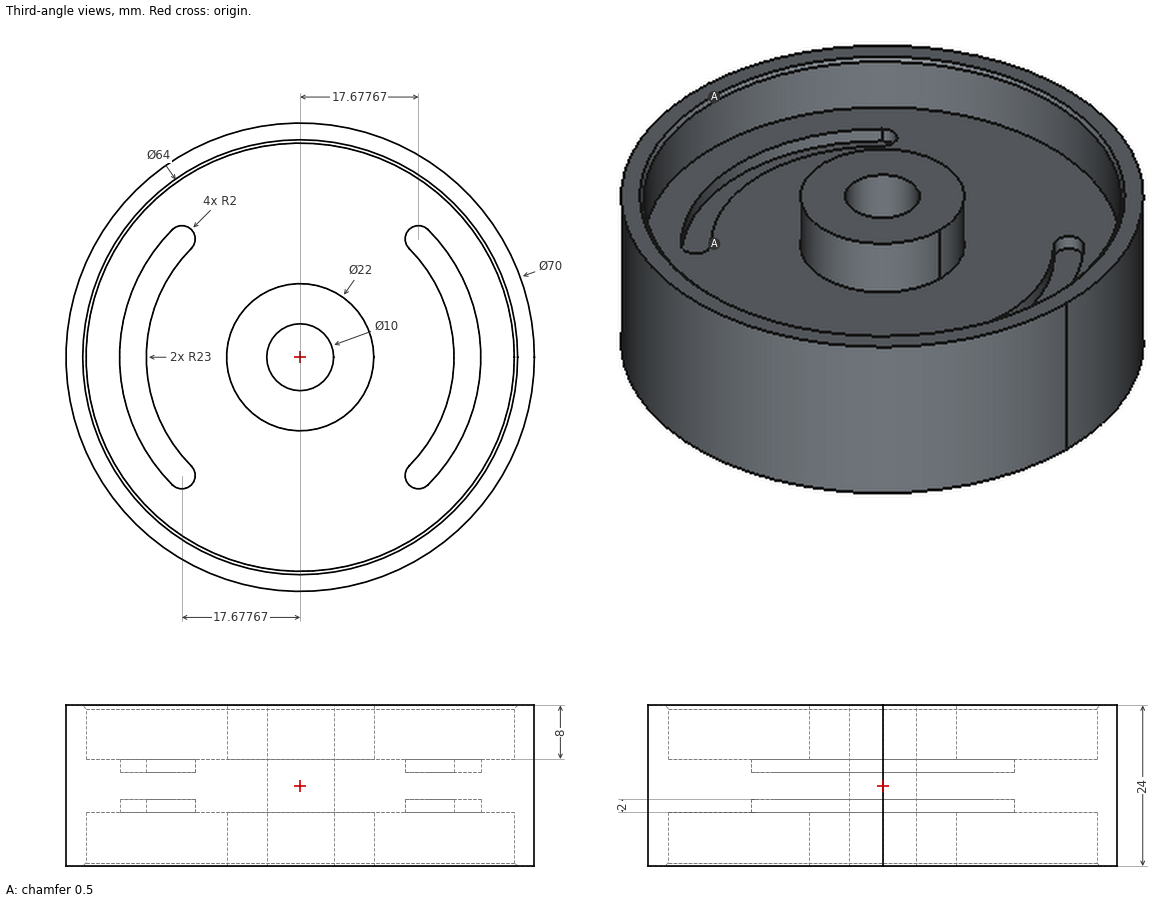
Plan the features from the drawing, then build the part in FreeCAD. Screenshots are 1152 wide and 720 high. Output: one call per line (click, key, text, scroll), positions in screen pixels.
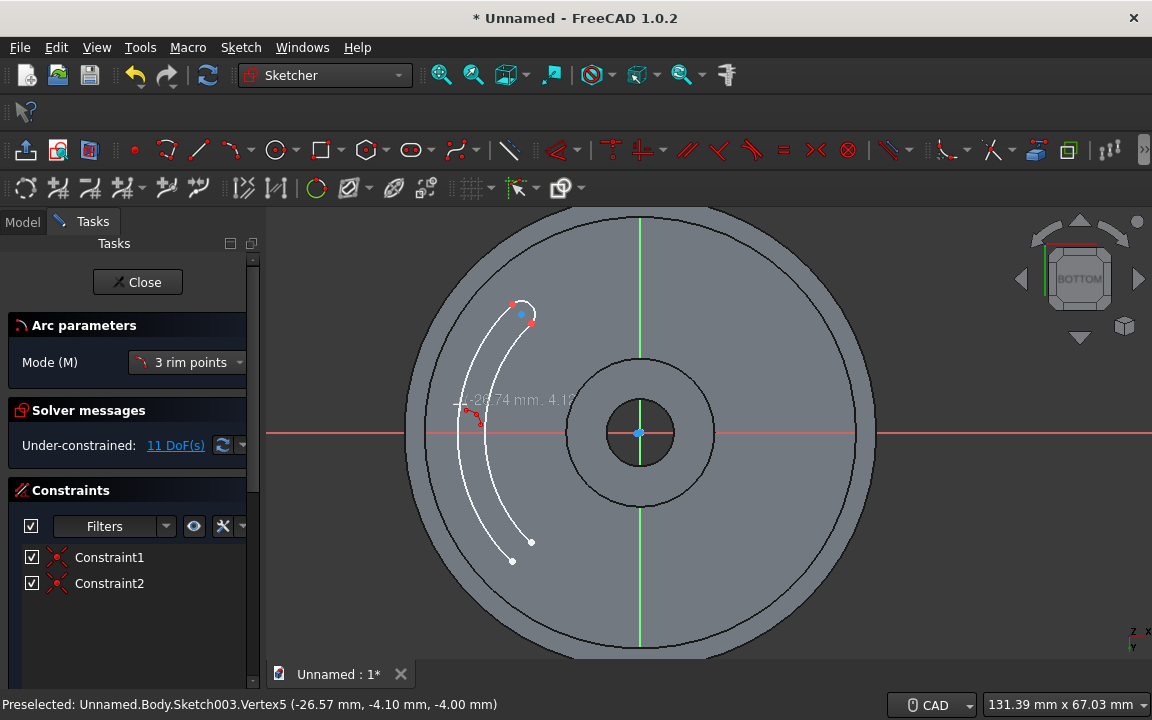
click(512, 562)
click(531, 543)
click(531, 561)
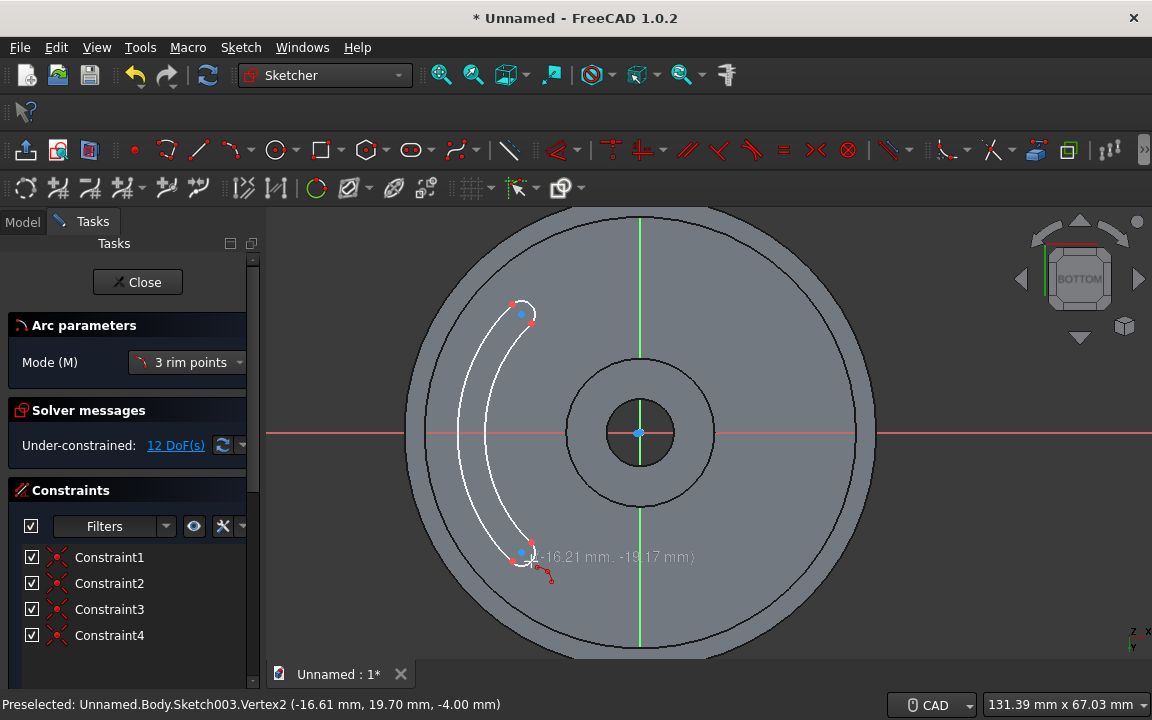
click(750, 323)
click(750, 542)
click(793, 457)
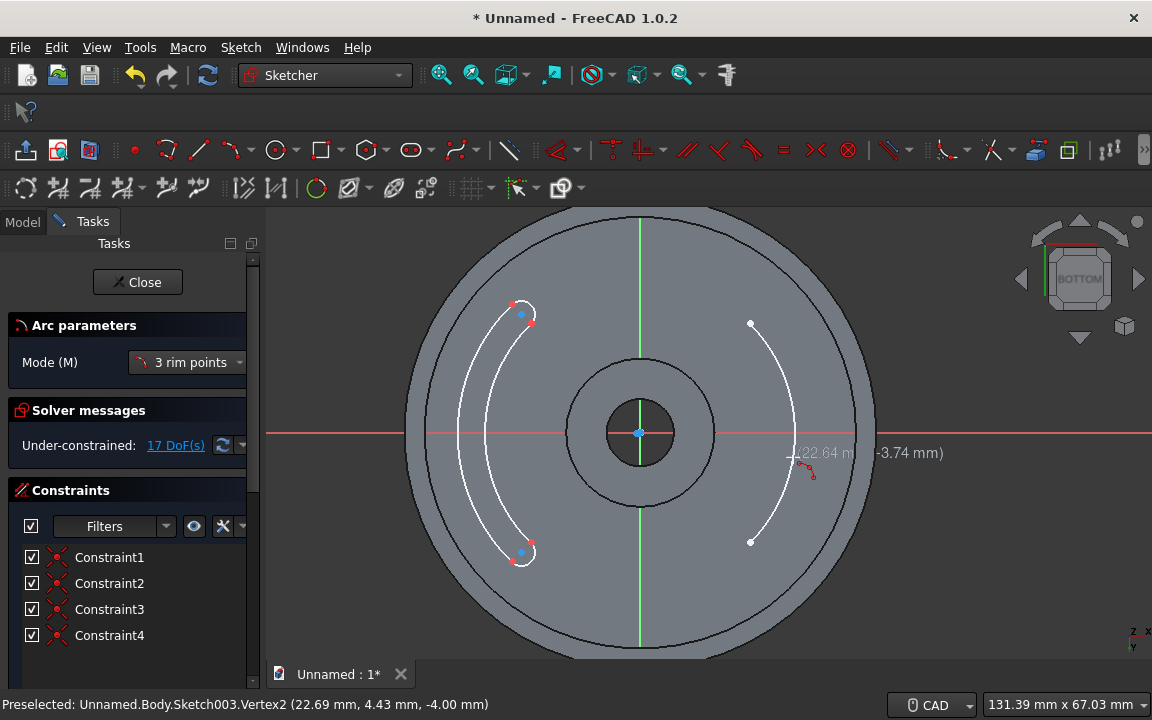
click(750, 543)
click(769, 561)
click(750, 561)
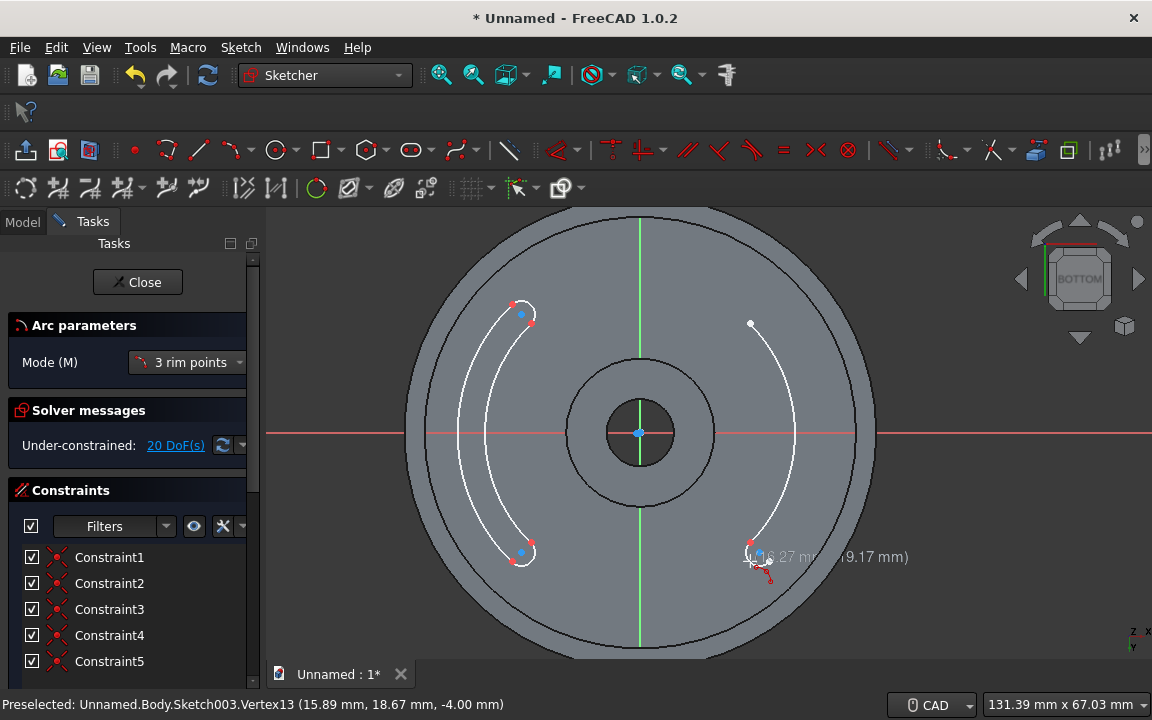
click(769, 562)
click(769, 304)
click(820, 461)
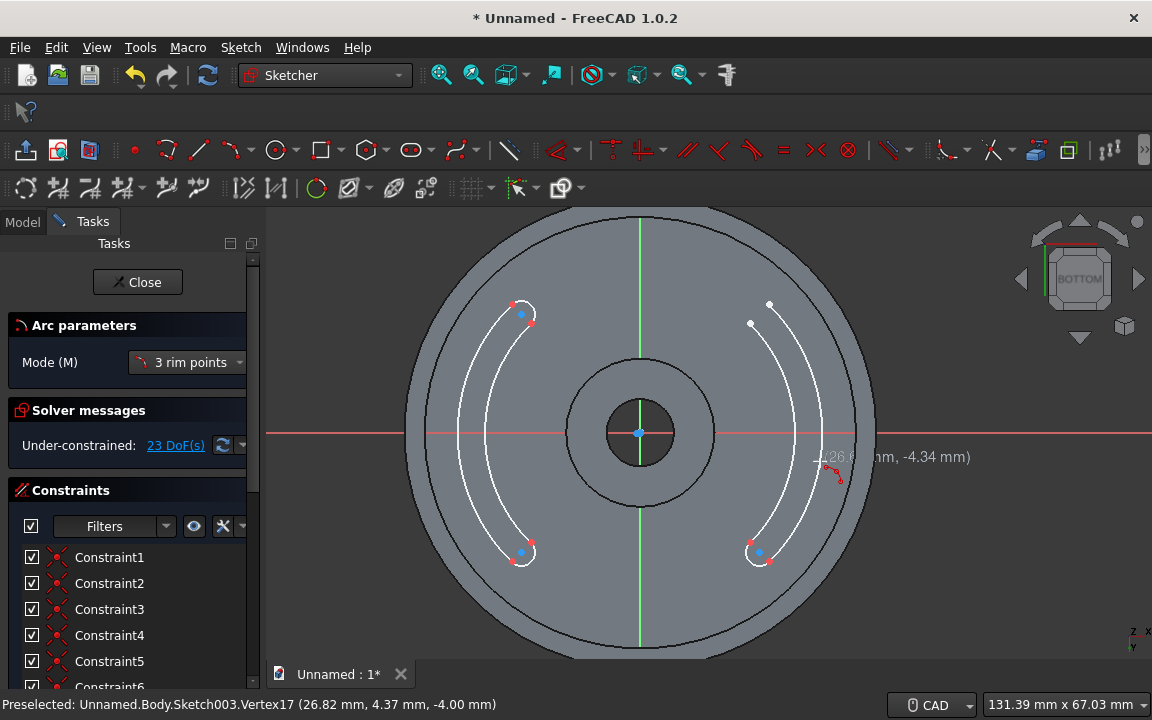
click(769, 305)
click(750, 324)
click(750, 304)
key(Escape)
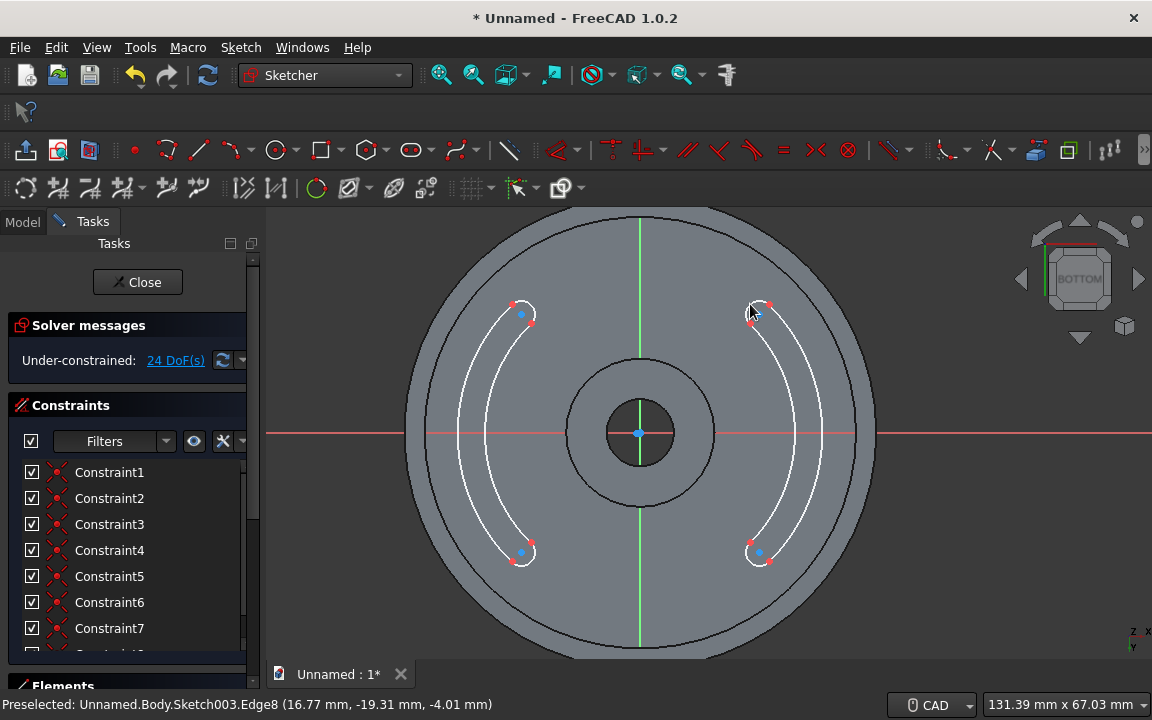
click(493, 386)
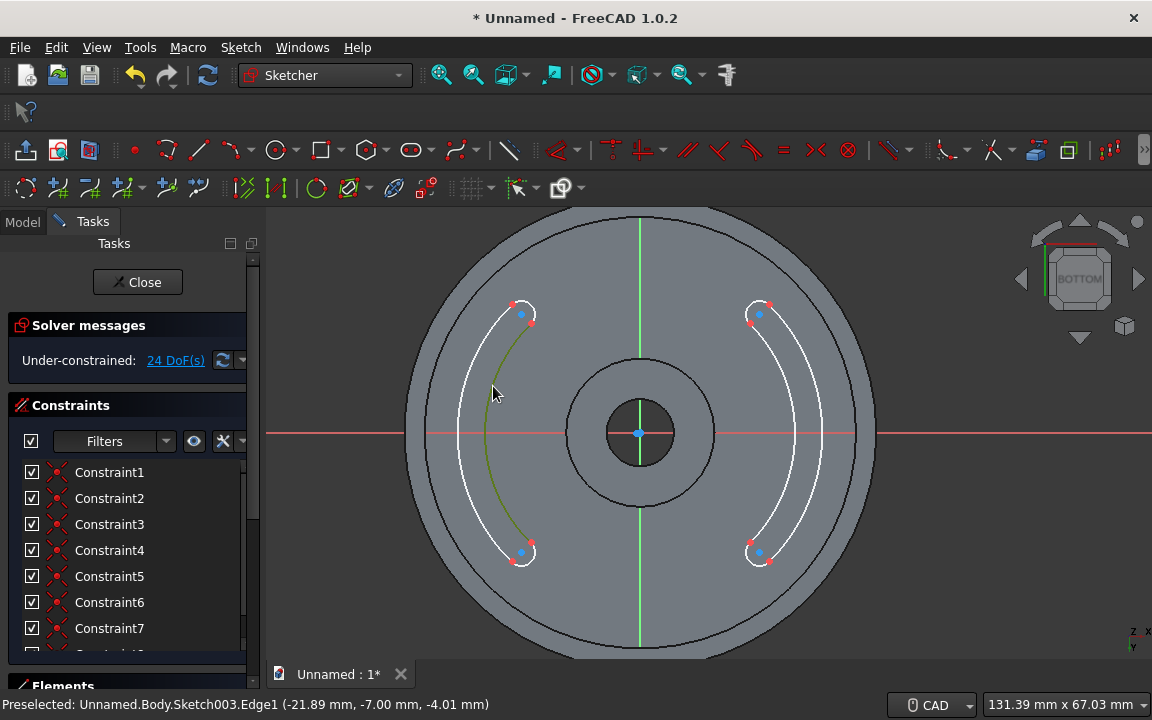
click(535, 312)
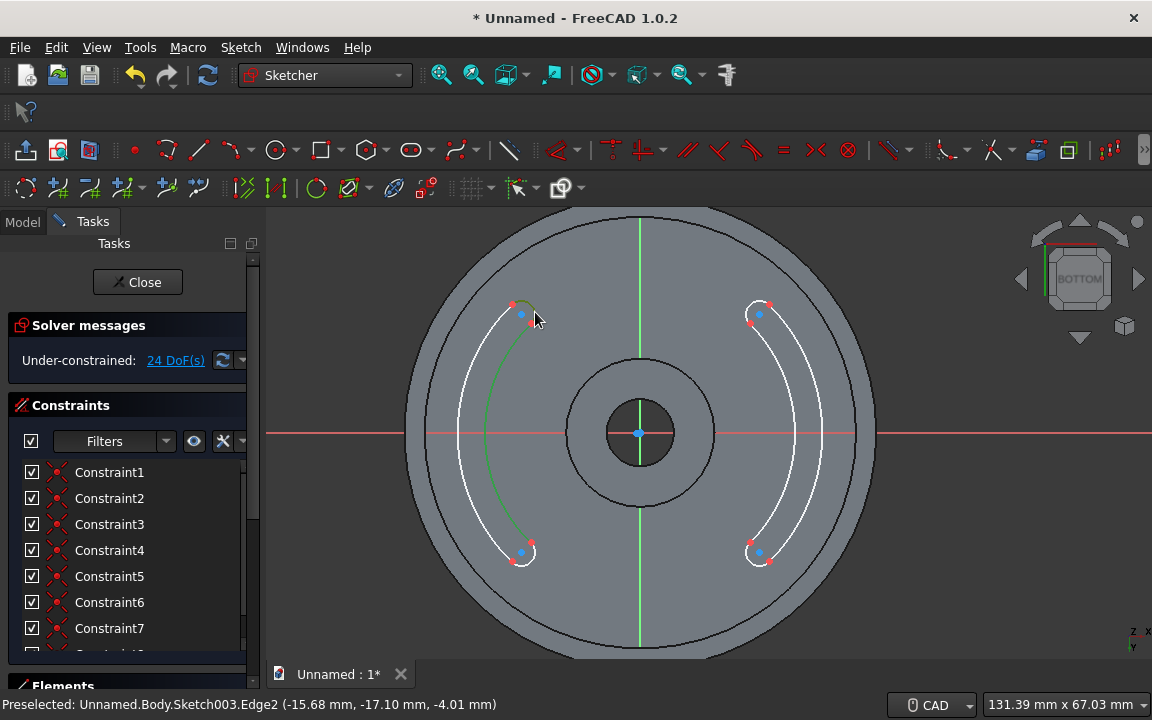
key(t)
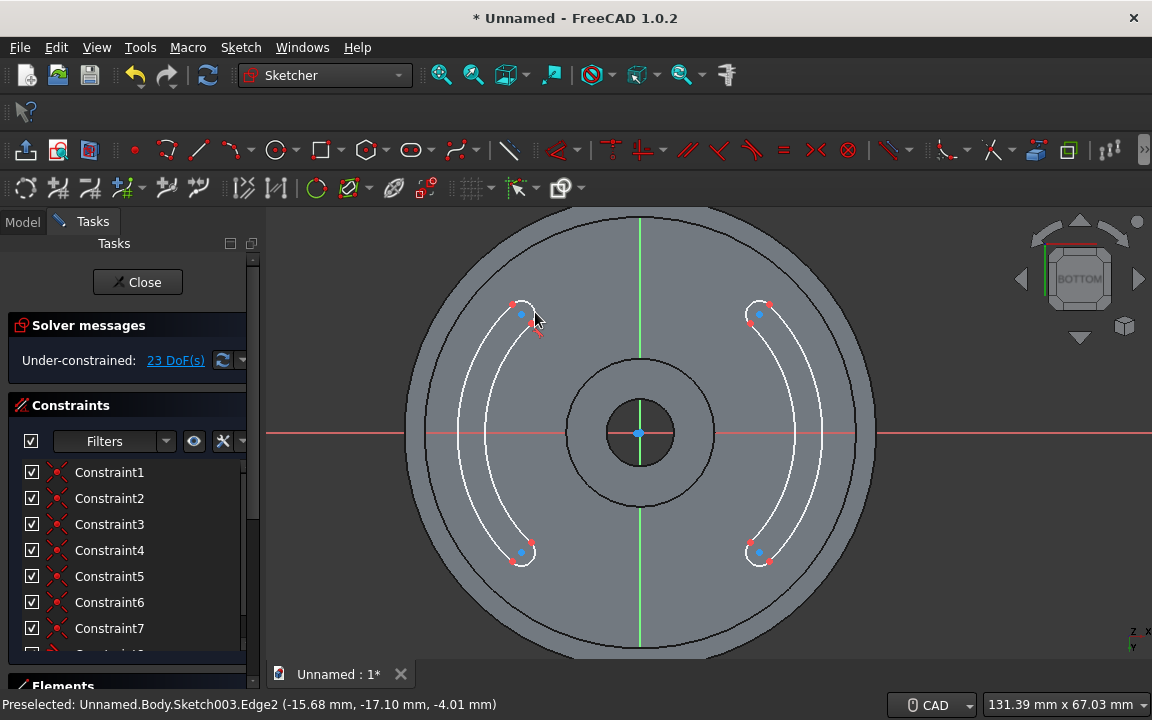
click(493, 386)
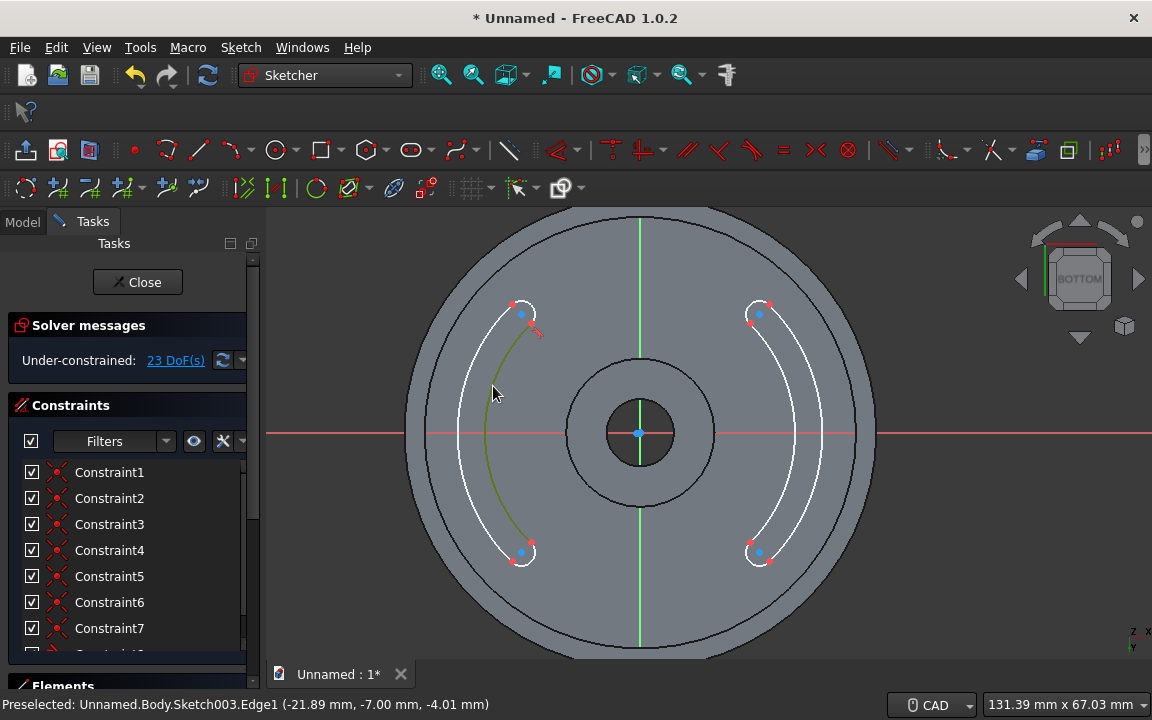
click(524, 566)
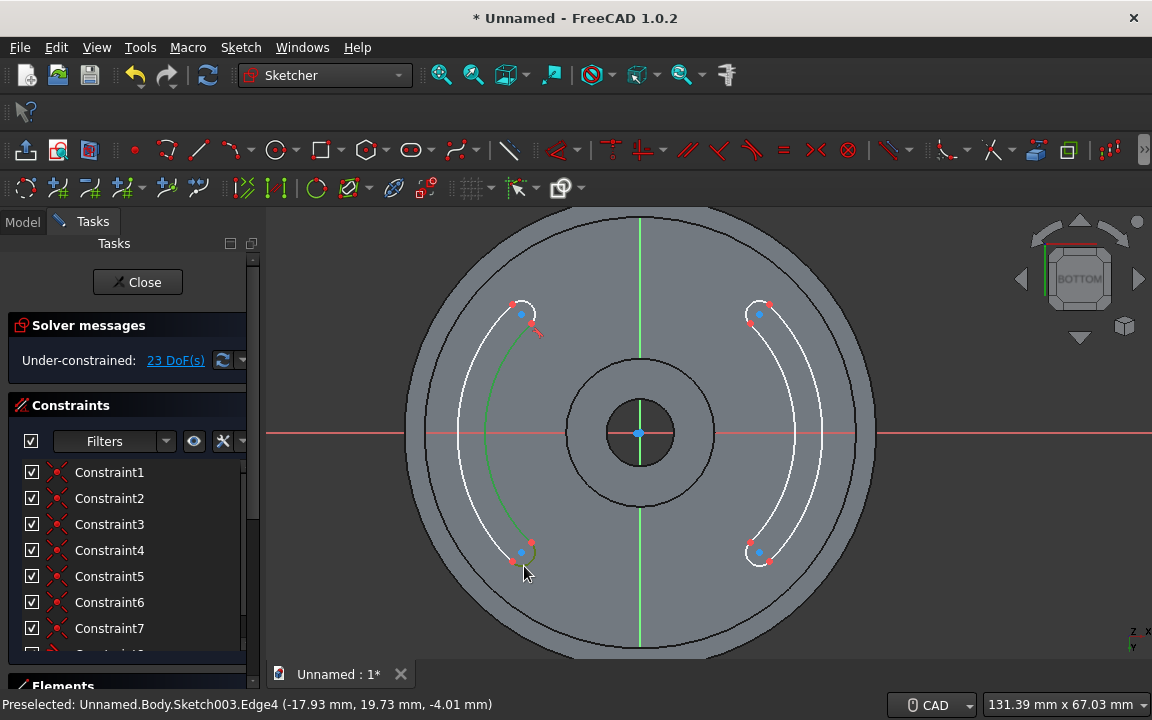
key(t)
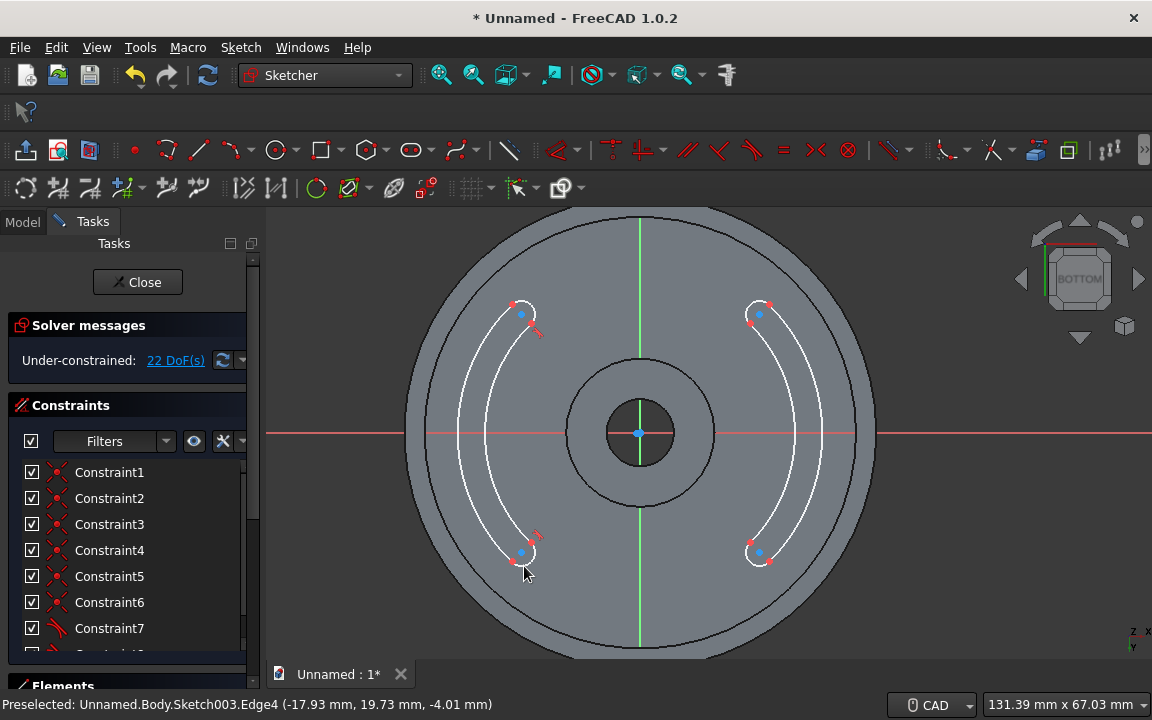
click(535, 312)